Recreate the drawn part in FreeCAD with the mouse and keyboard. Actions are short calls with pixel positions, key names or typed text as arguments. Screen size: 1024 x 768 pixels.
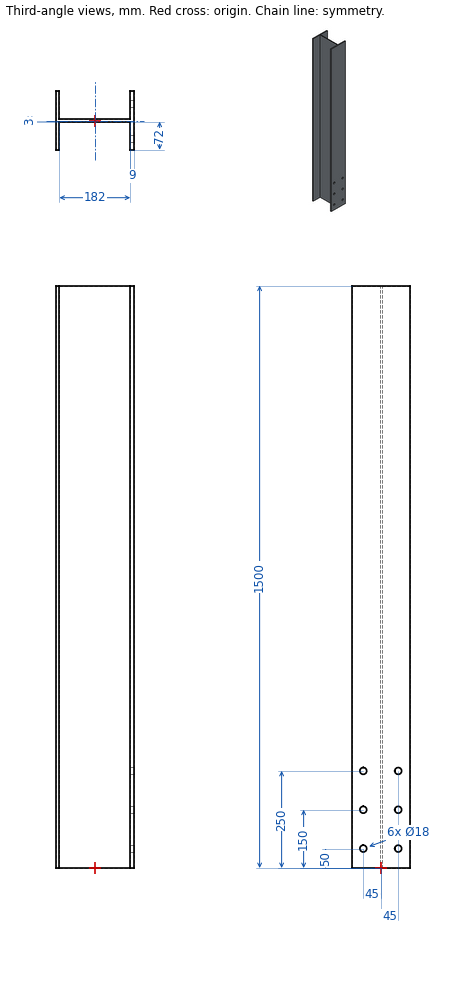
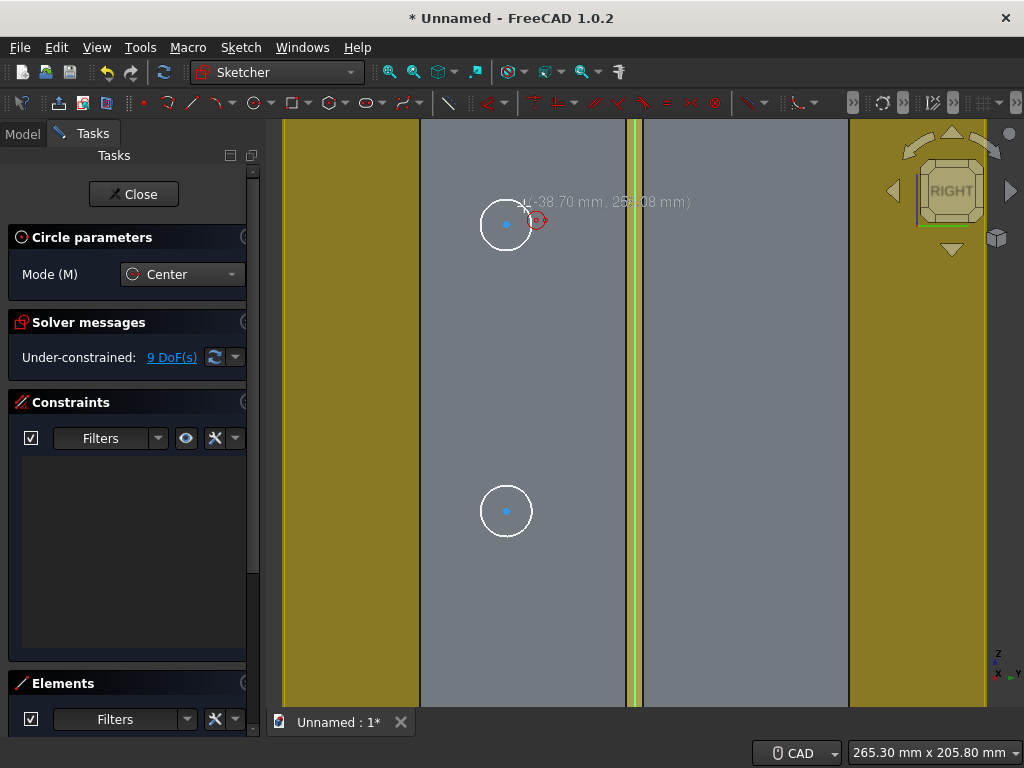
click(763, 224)
click(781, 206)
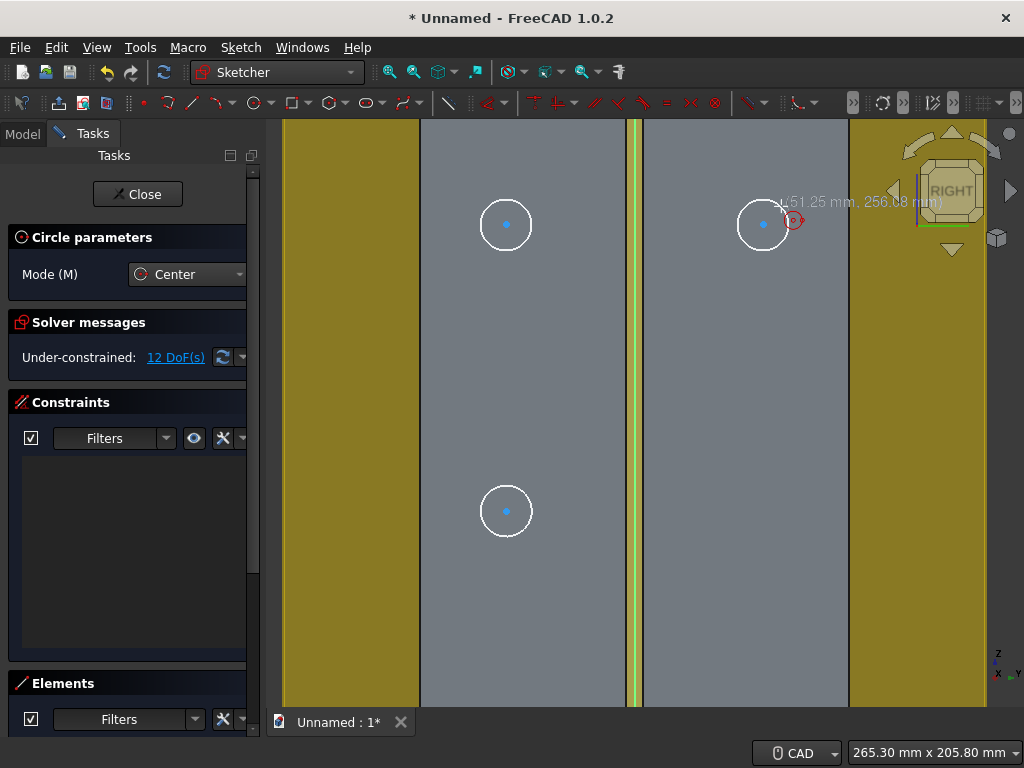
click(763, 510)
click(781, 492)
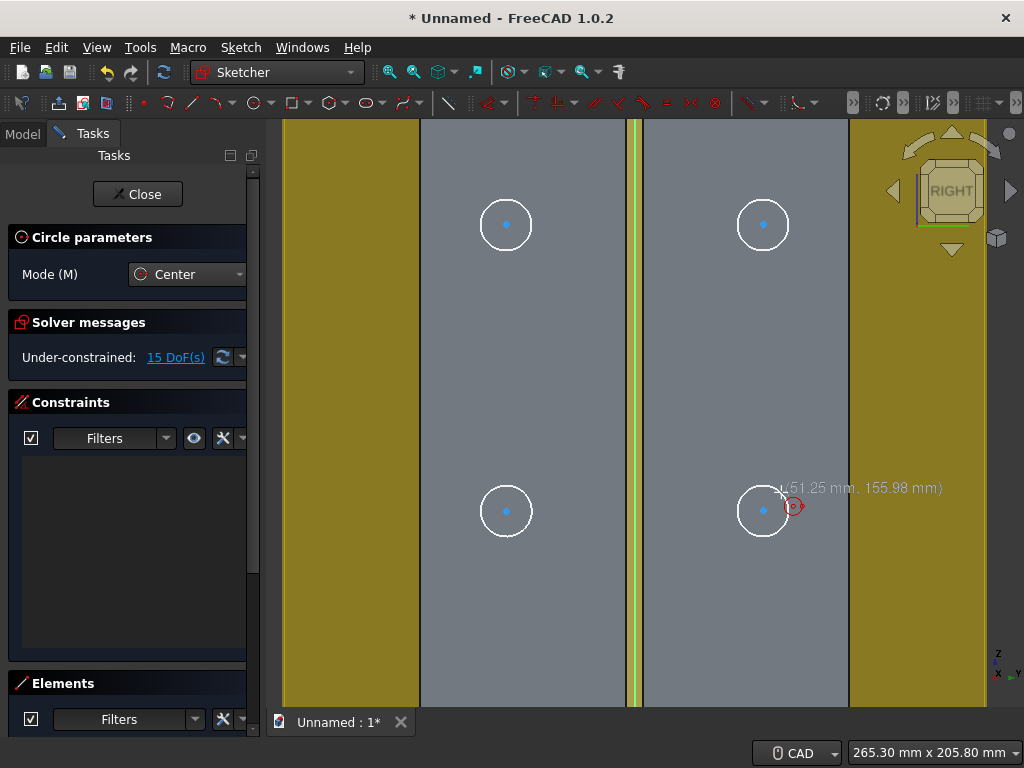
scroll(506, 224, down, 3)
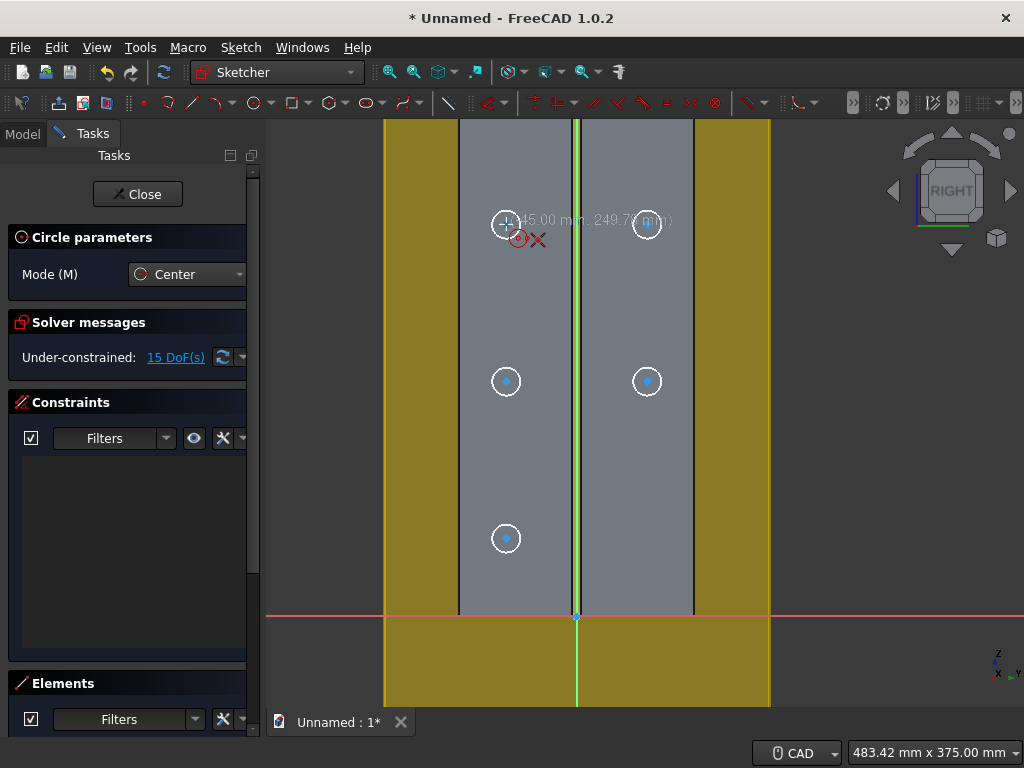
scroll(647, 538, up, 3)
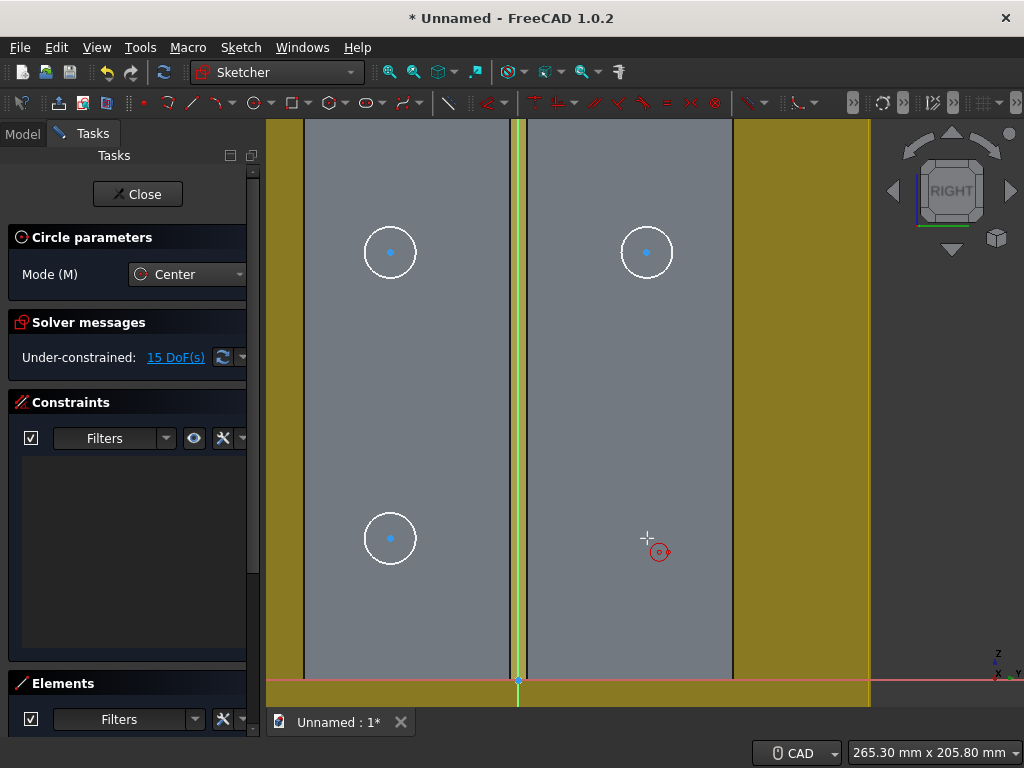
click(647, 537)
click(665, 519)
key(Escape)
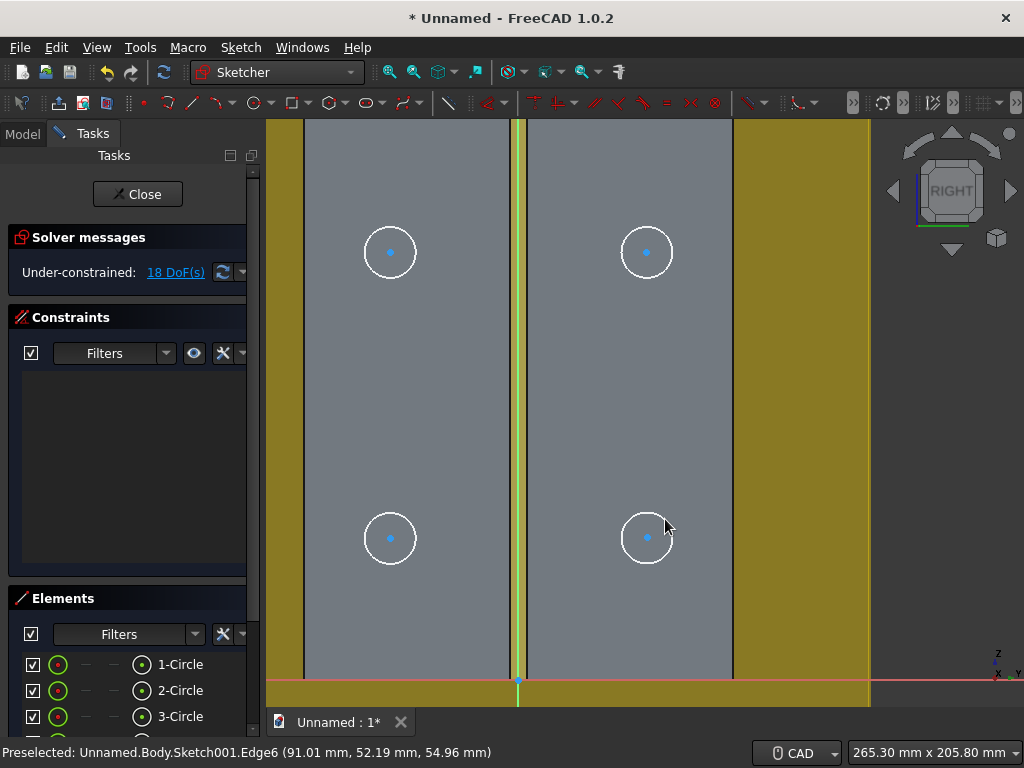
click(408, 520)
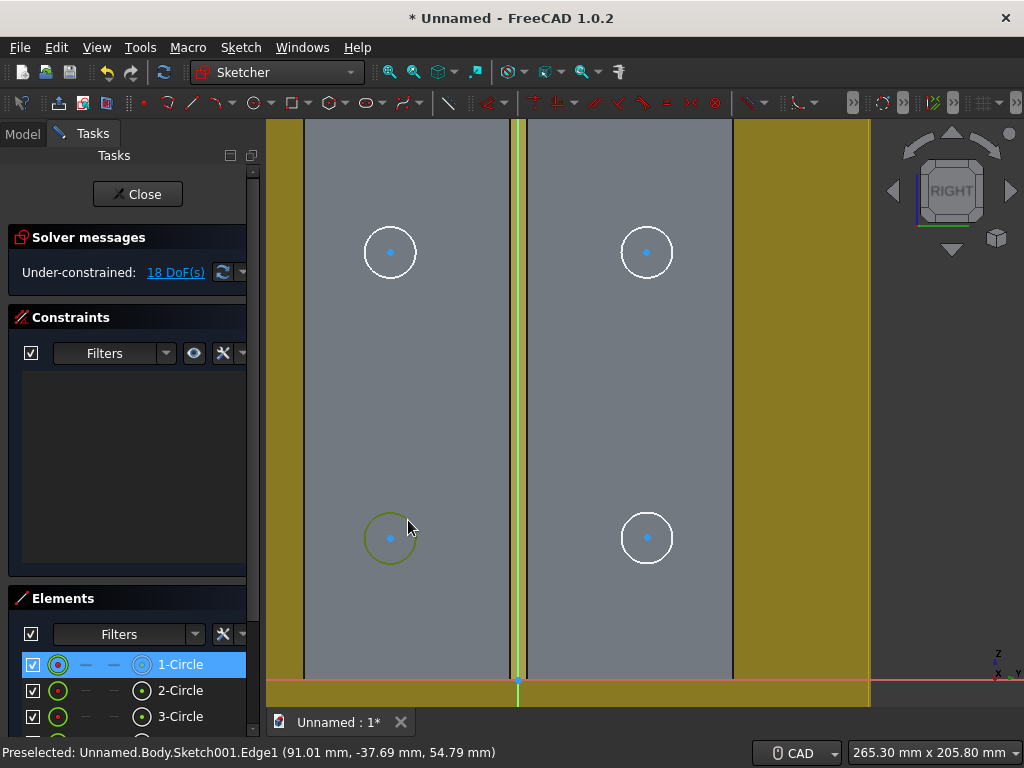
click(408, 234)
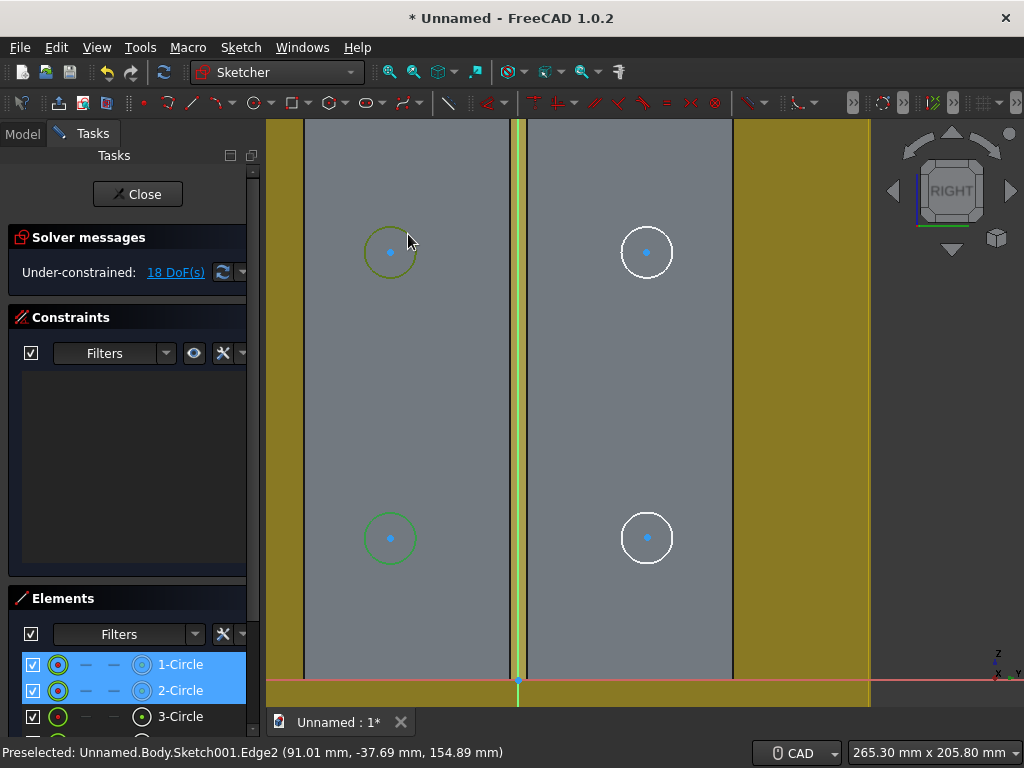
scroll(647, 538, down, 3)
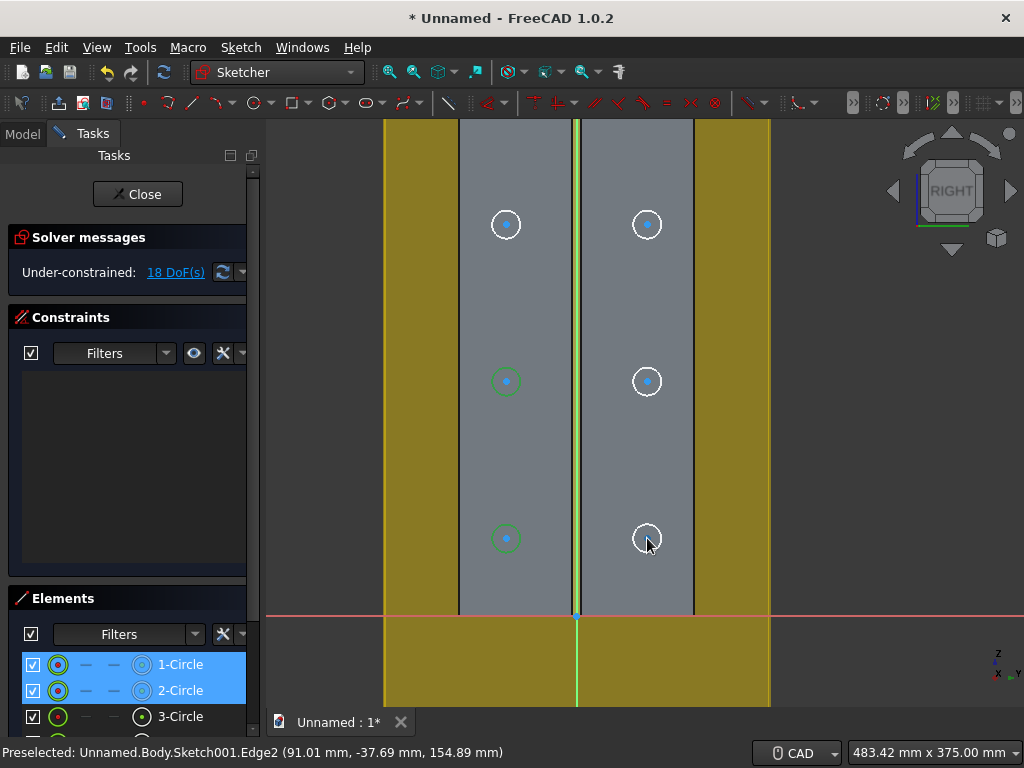
click(516, 215)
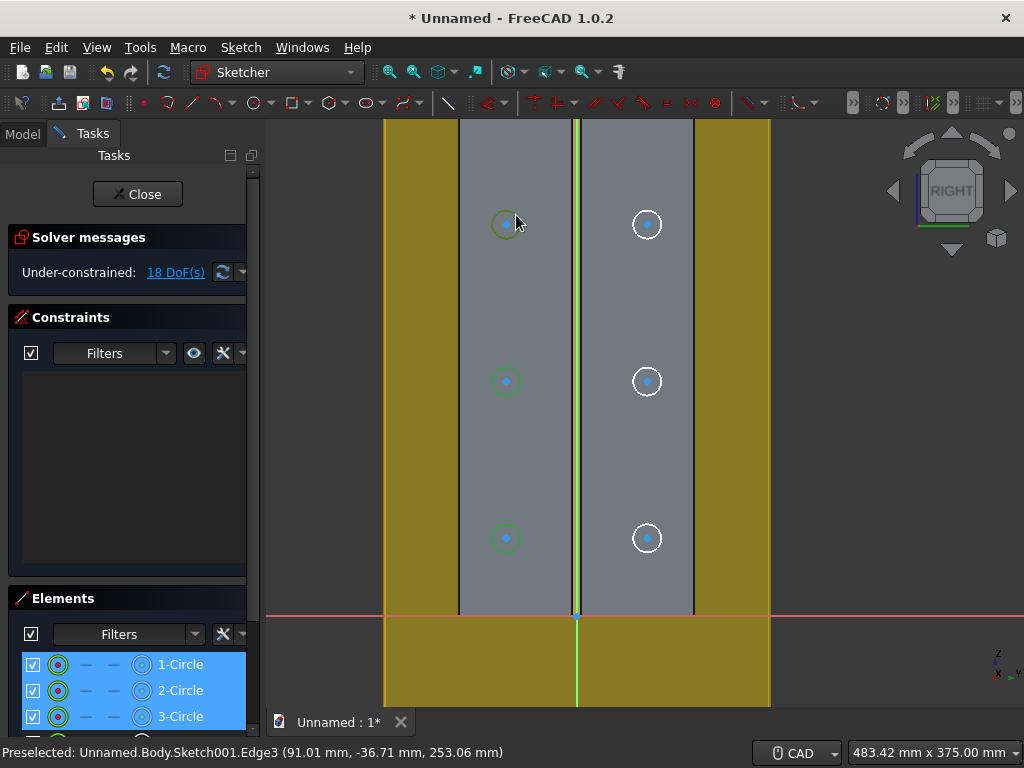
click(657, 215)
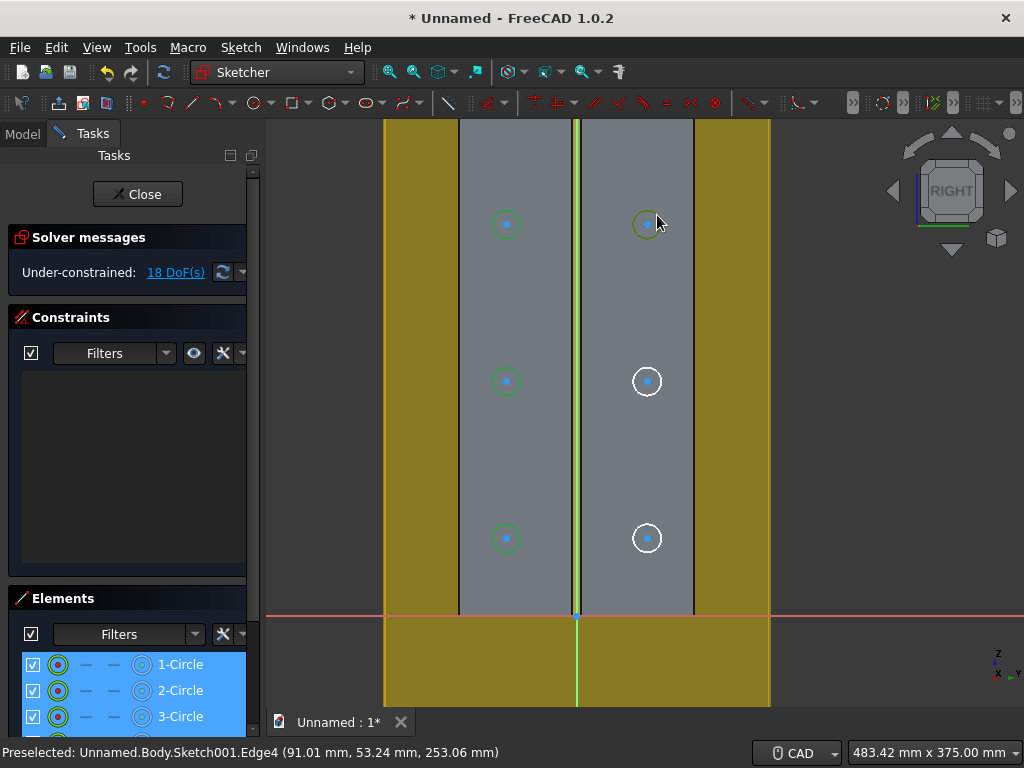
click(657, 372)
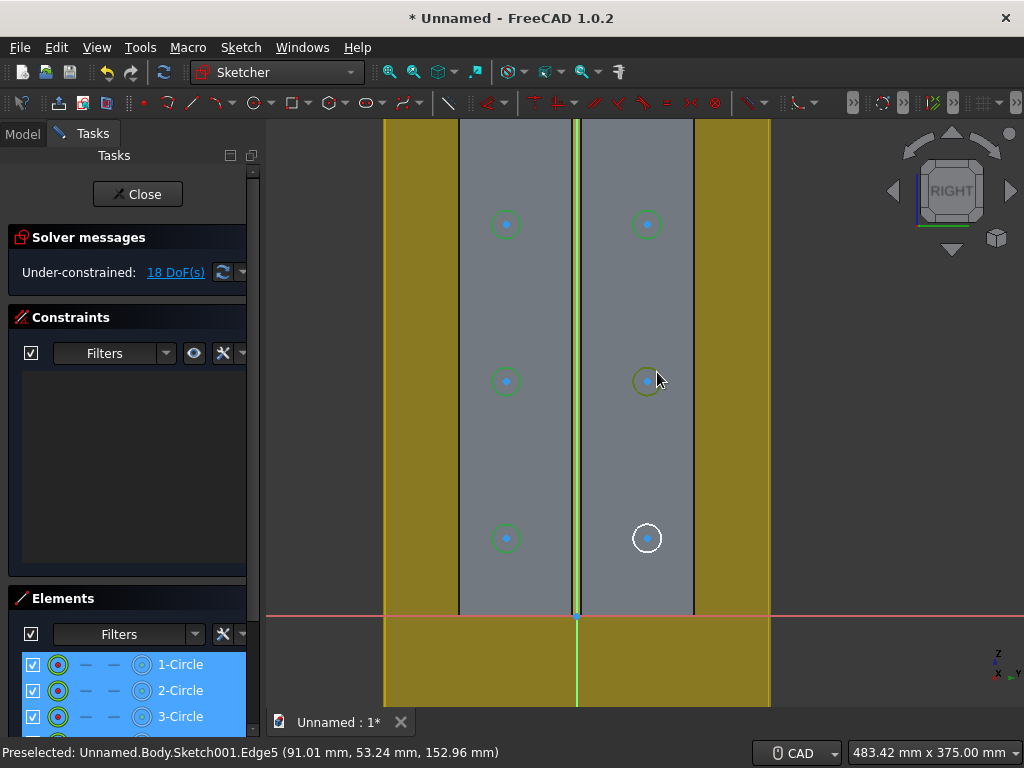
click(657, 528)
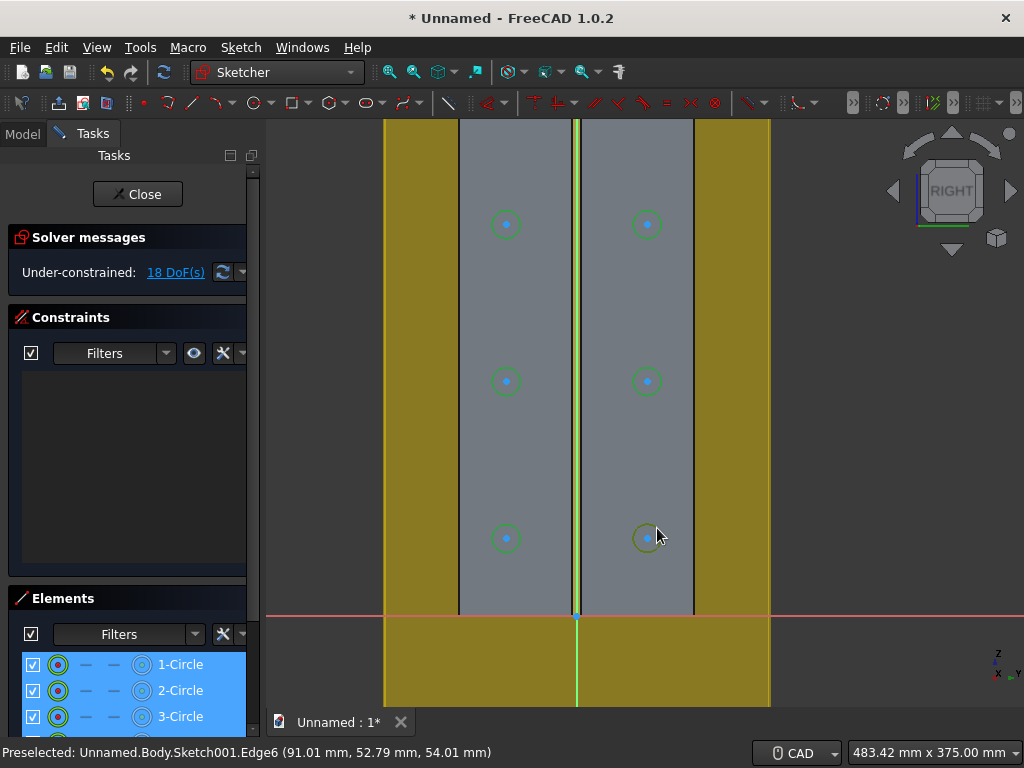
key(e)